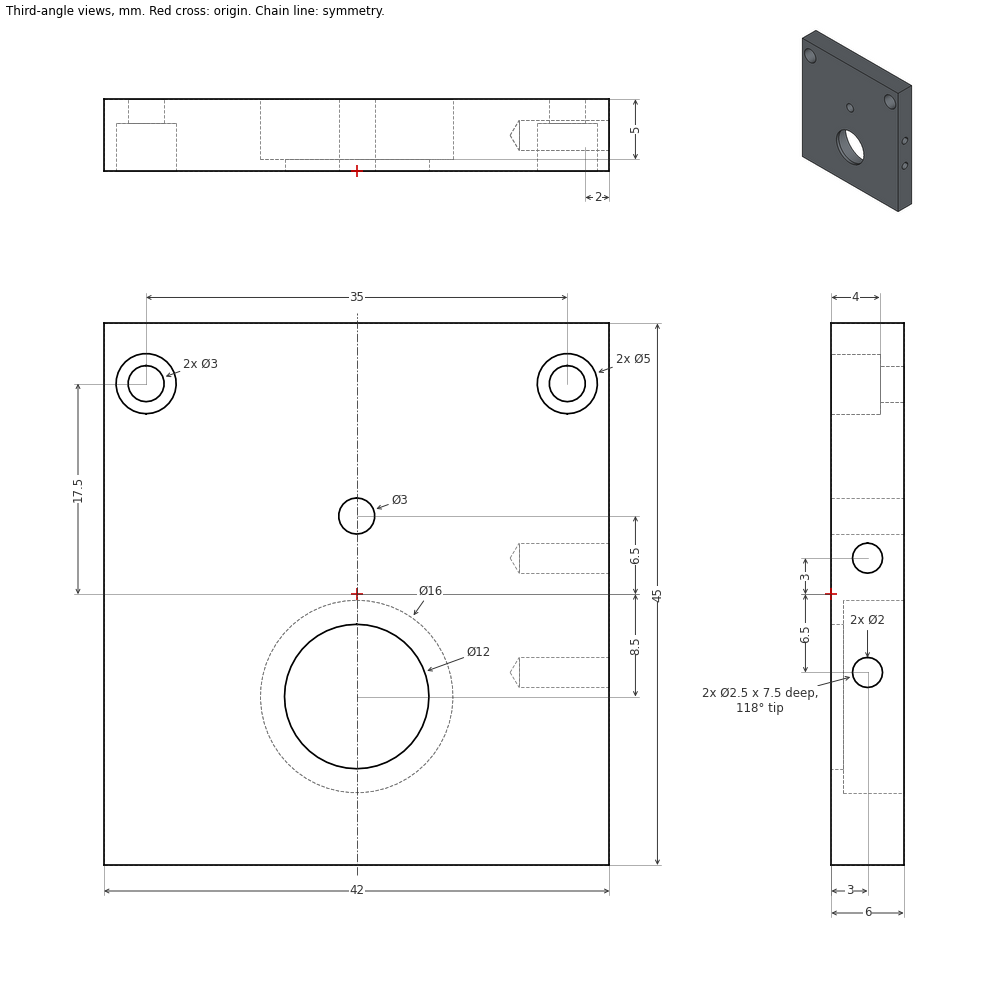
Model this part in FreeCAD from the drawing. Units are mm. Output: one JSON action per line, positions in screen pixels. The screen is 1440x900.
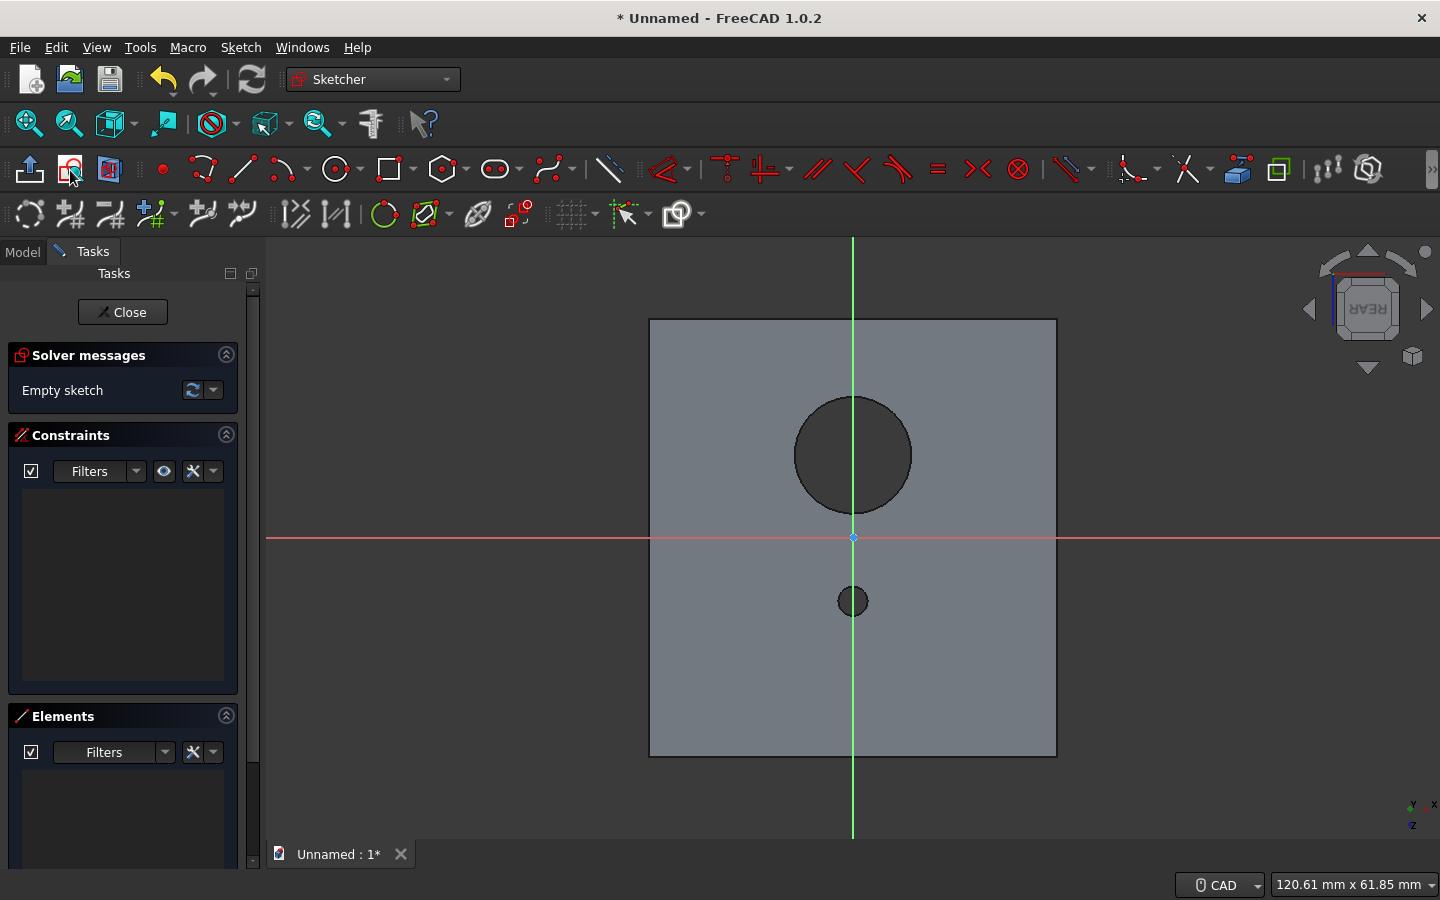
{"action": "scroll", "coordinate": [909, 392], "scroll_direction": "up", "scroll_amount": 4}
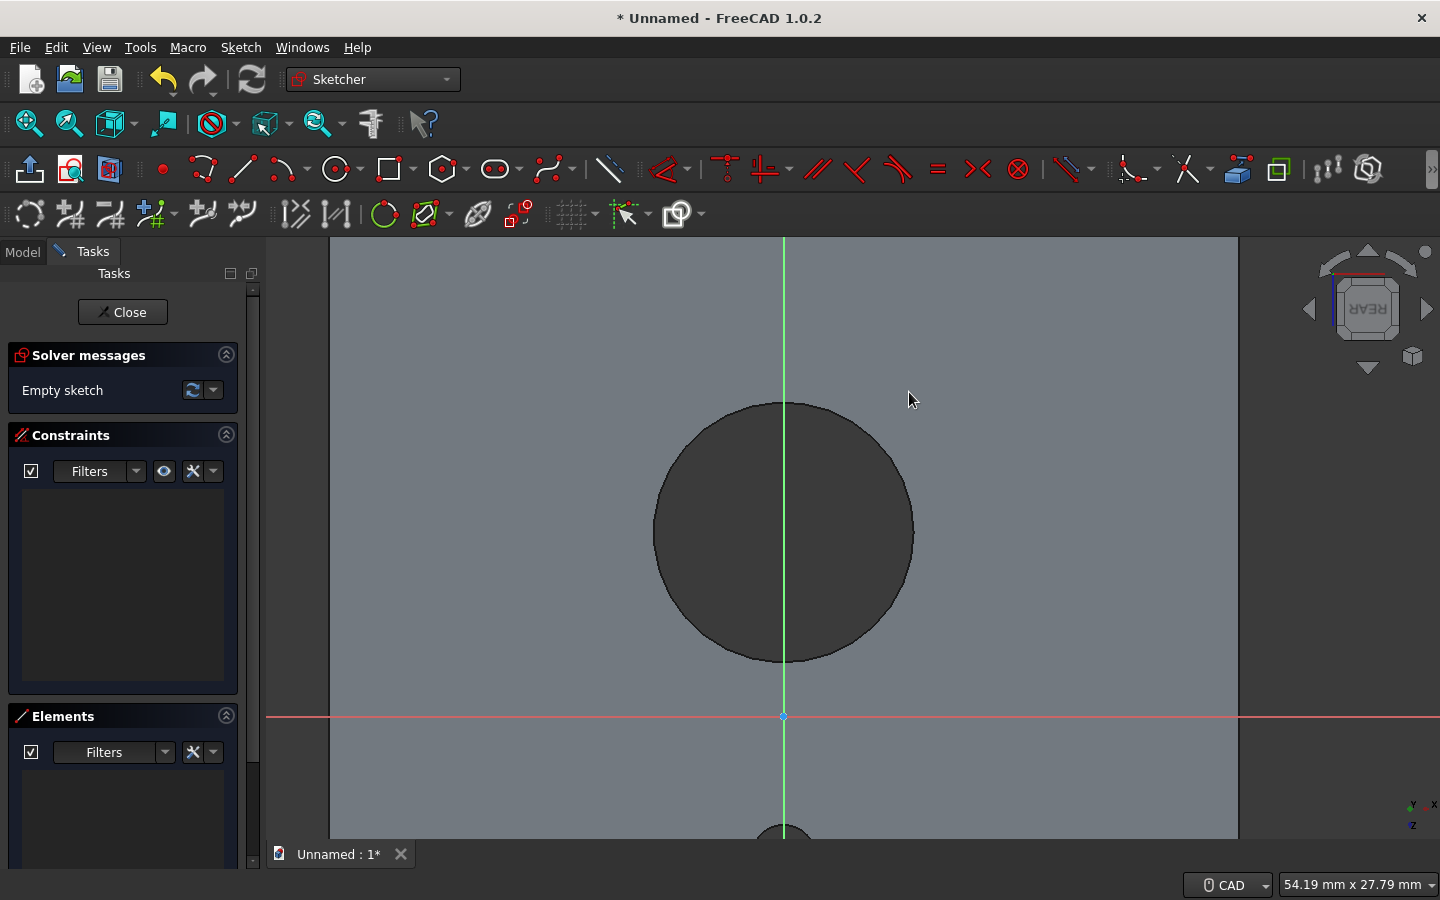
{"action": "key", "text": "g c"}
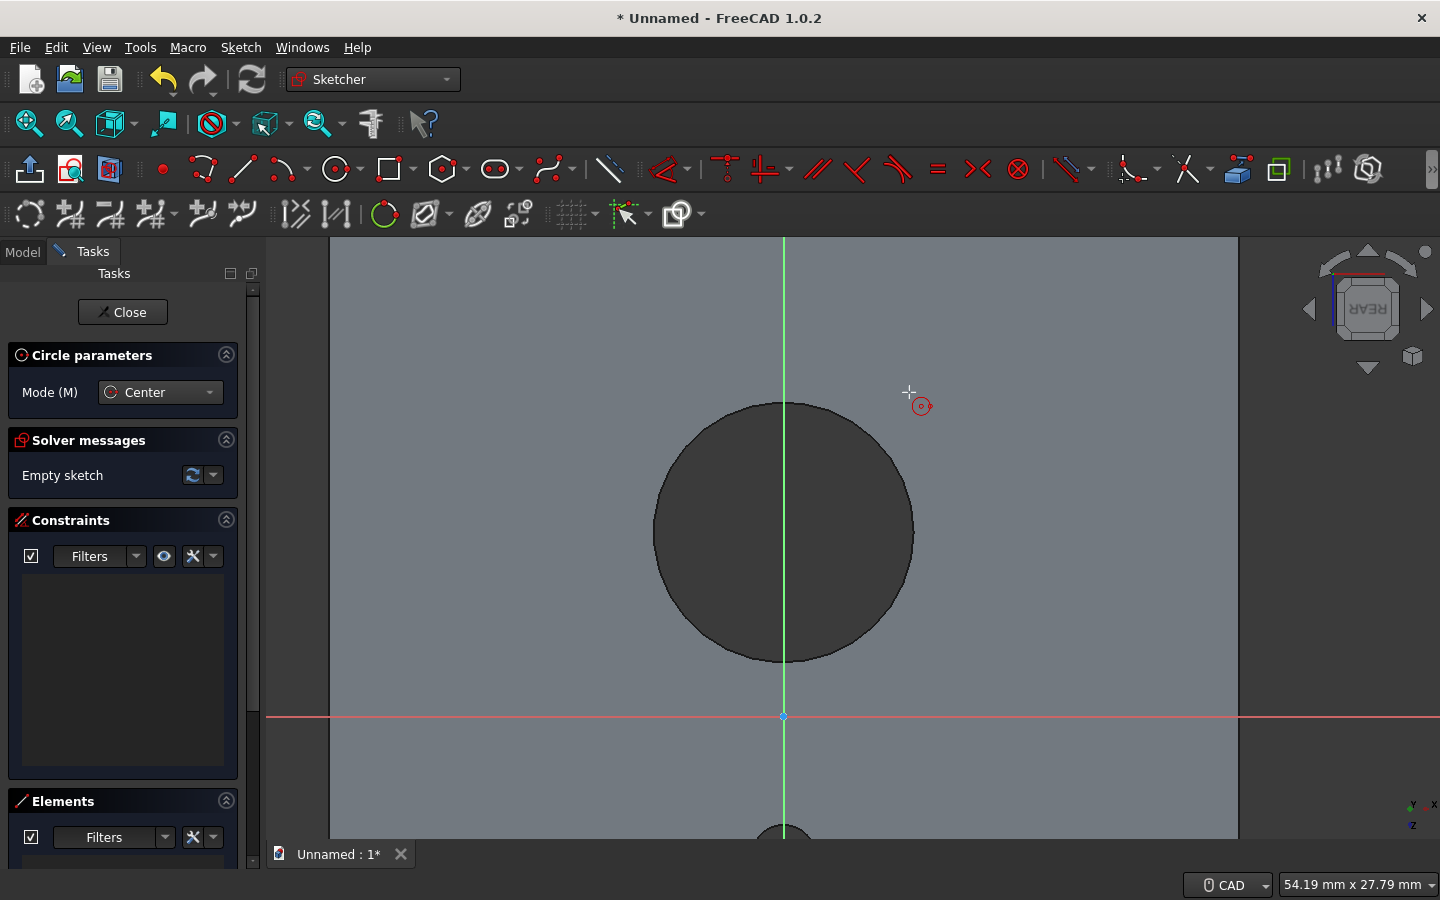
{"action": "left_click", "coordinate": [784, 532]}
{"action": "mouse_move", "coordinate": [906, 410]}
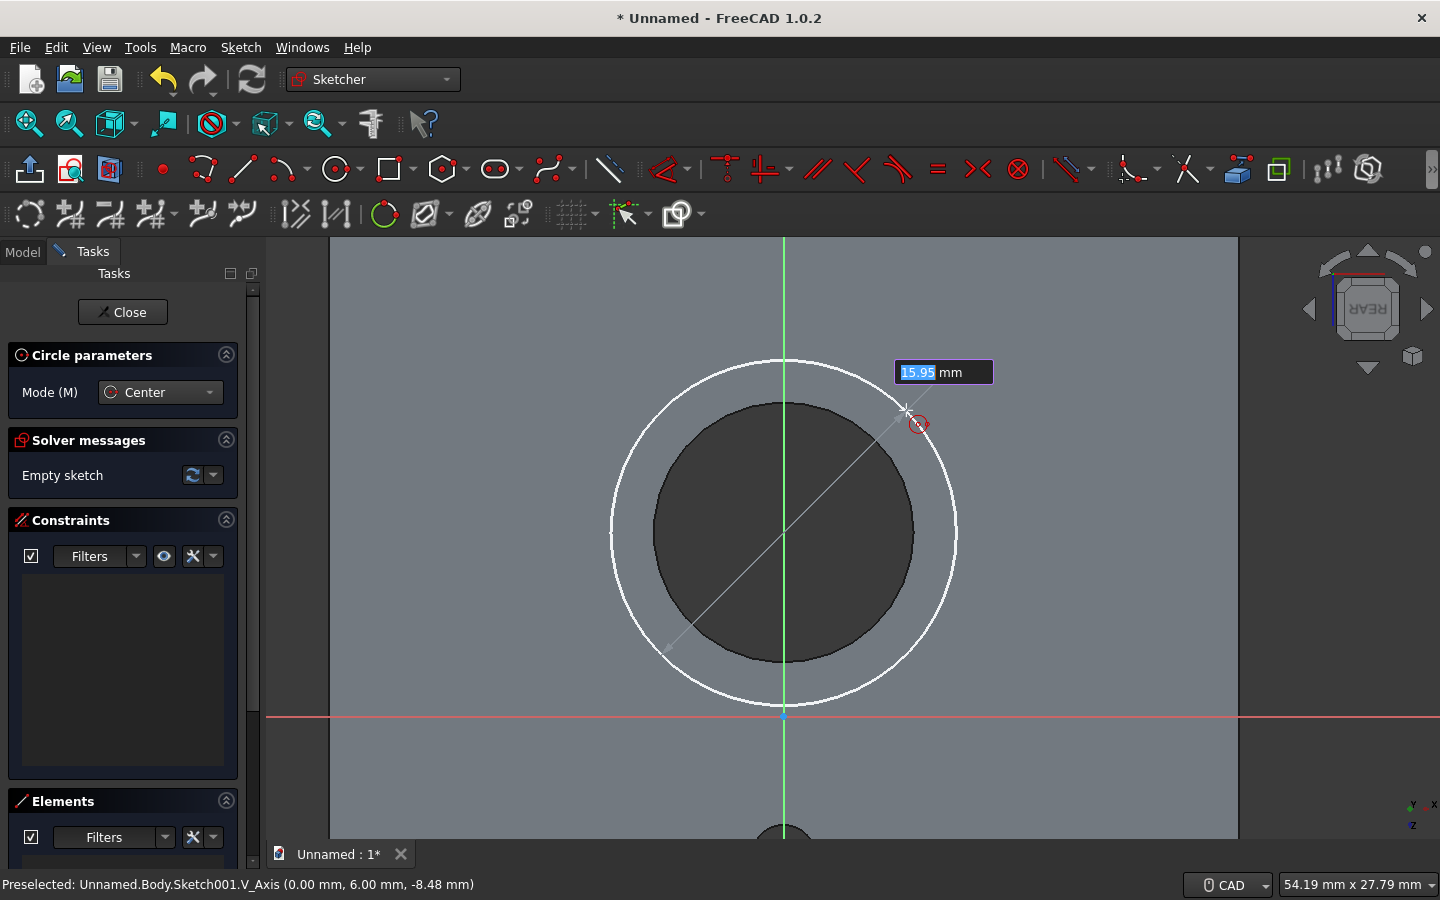
{"action": "type", "text": "16"}
{"action": "key", "text": "Return"}
{"action": "key", "text": "Escape"}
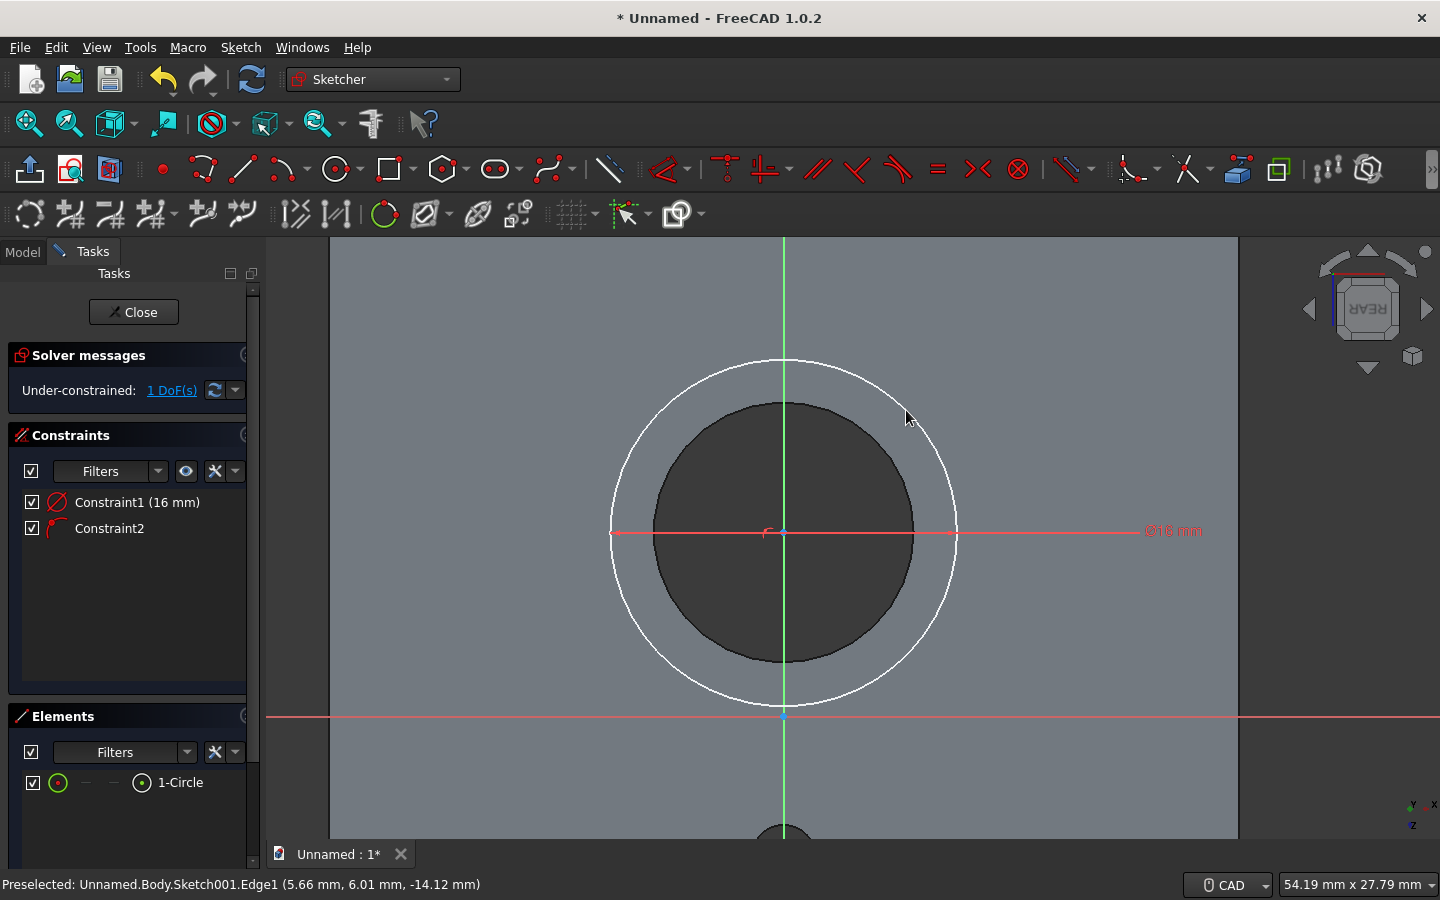
{"action": "key", "text": "d"}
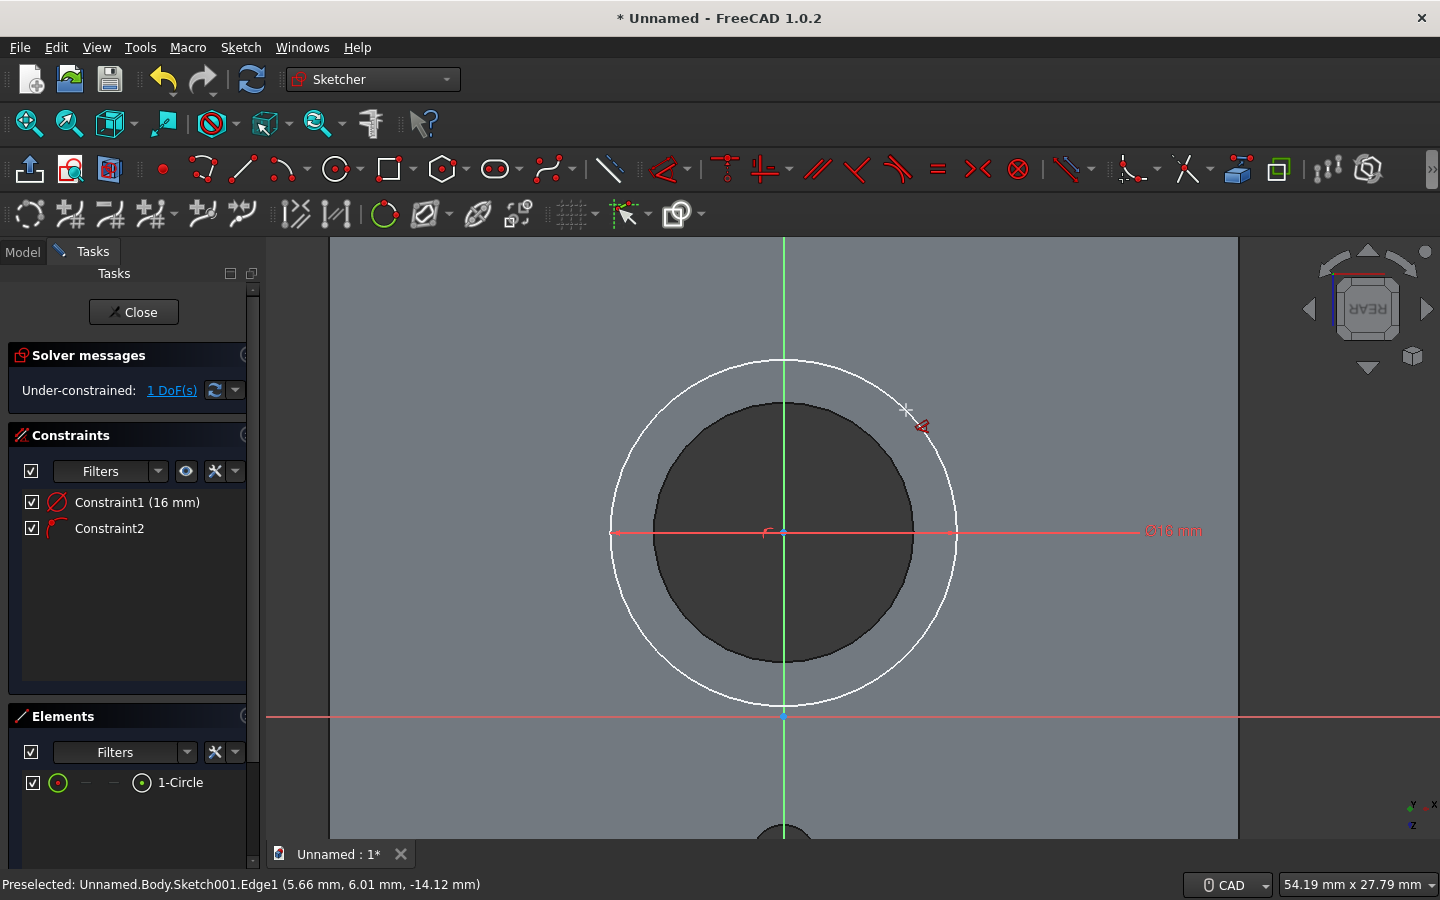
{"action": "left_click", "coordinate": [784, 533]}
{"action": "left_click", "coordinate": [818, 625]}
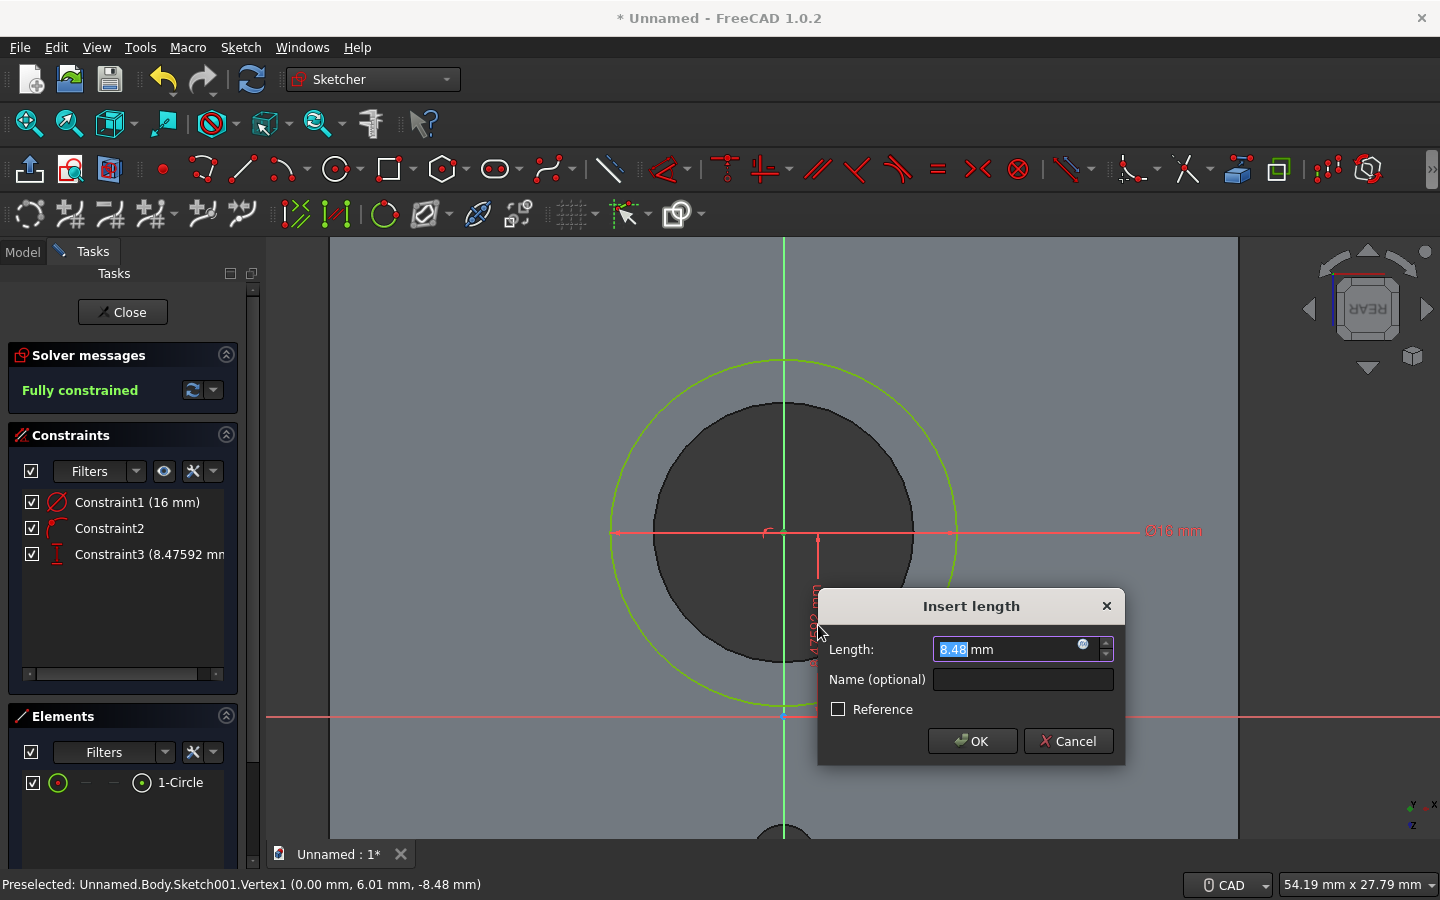
{"action": "type", "text": "8.5"}
{"action": "key", "text": "Return"}
{"action": "key", "text": "Escape"}